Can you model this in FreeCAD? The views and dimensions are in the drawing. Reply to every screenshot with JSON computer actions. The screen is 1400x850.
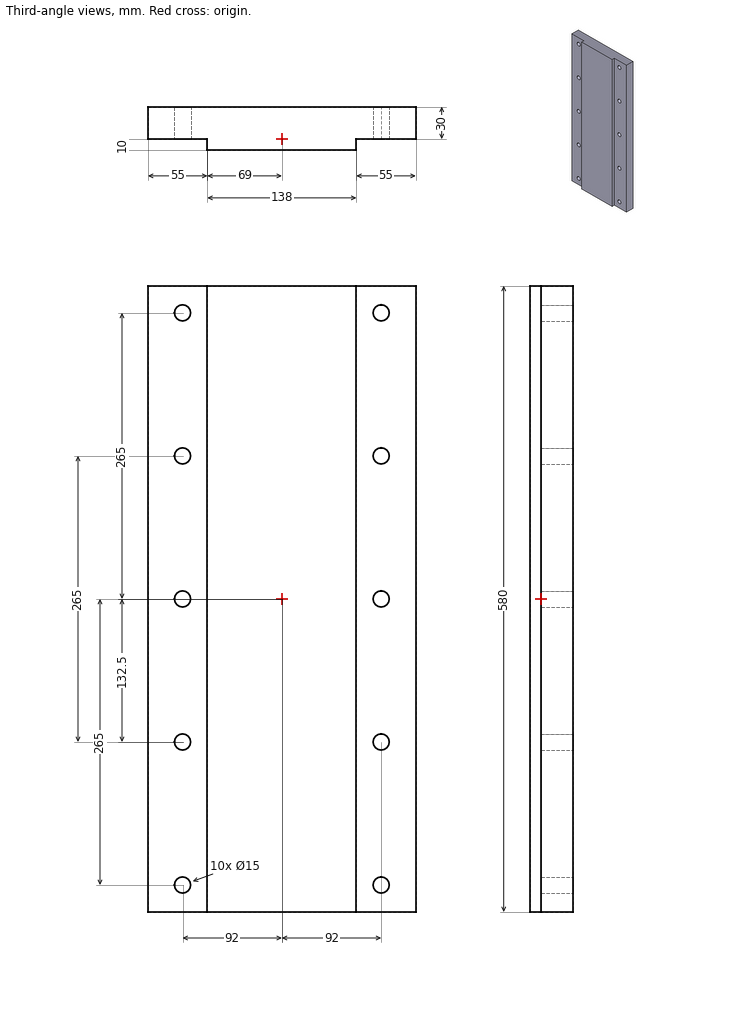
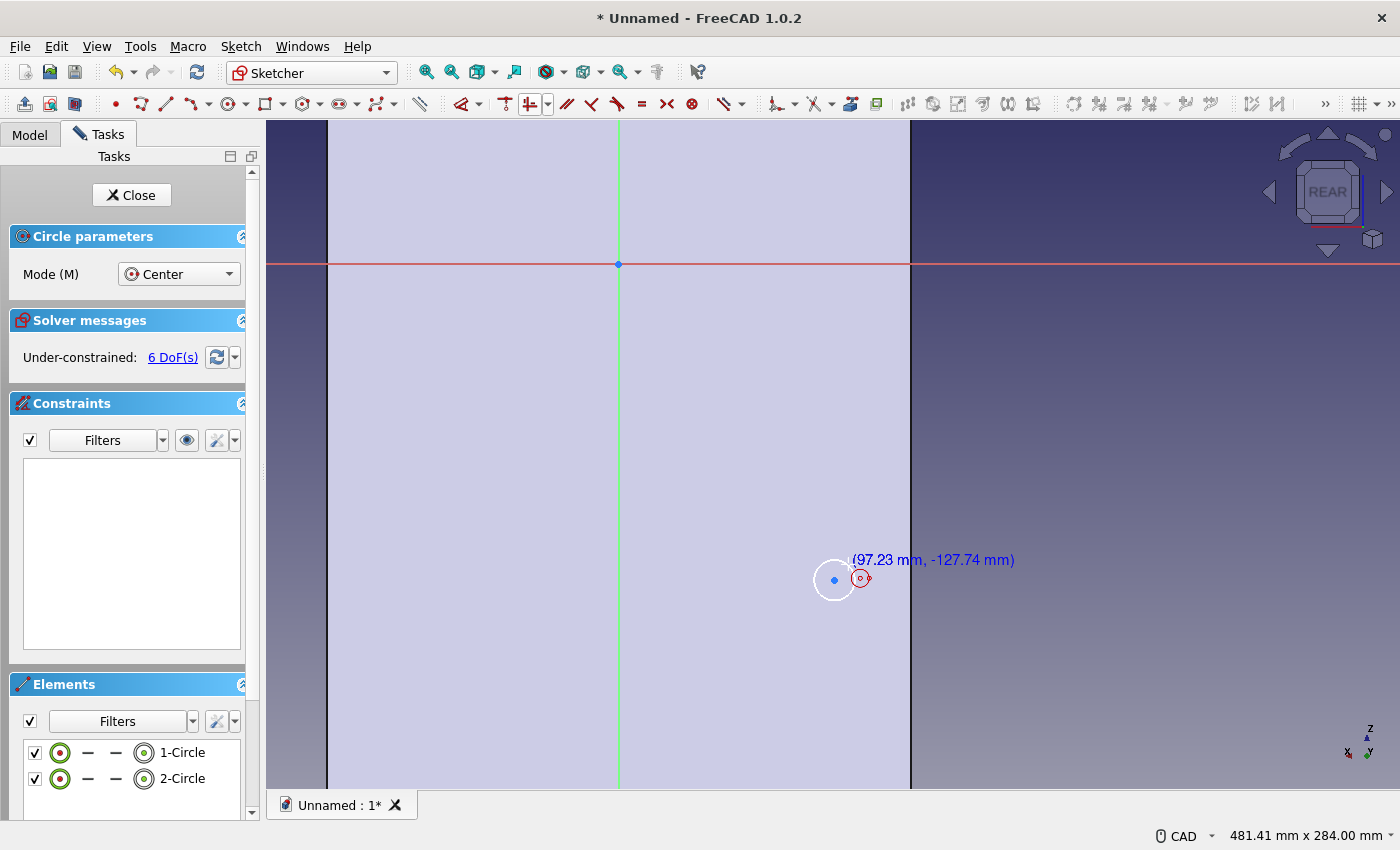
{"action": "scroll", "coordinate": [836, 264], "scroll_direction": "up", "scroll_amount": 2}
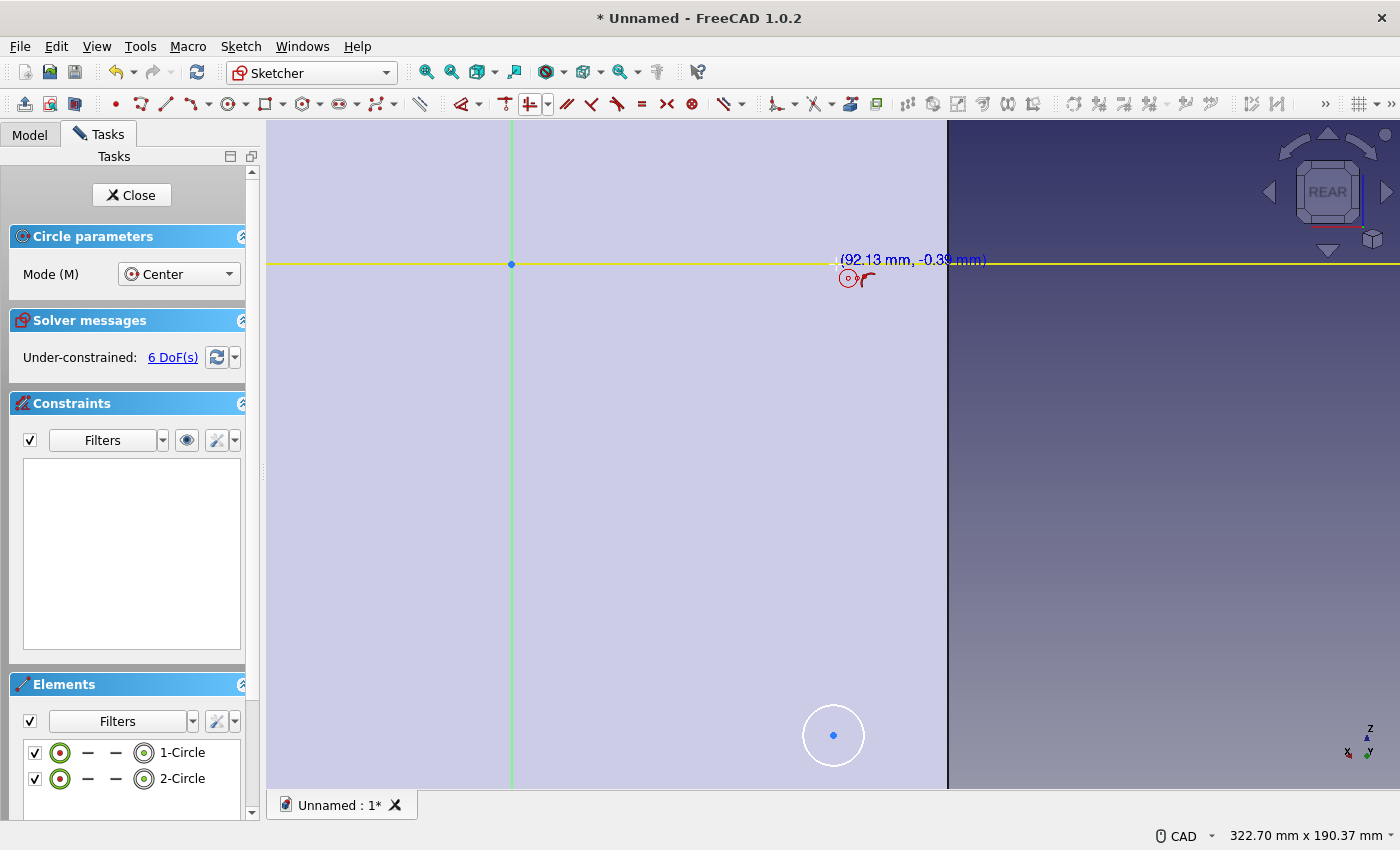
{"action": "scroll", "coordinate": [847, 517], "scroll_direction": "down", "scroll_amount": 7}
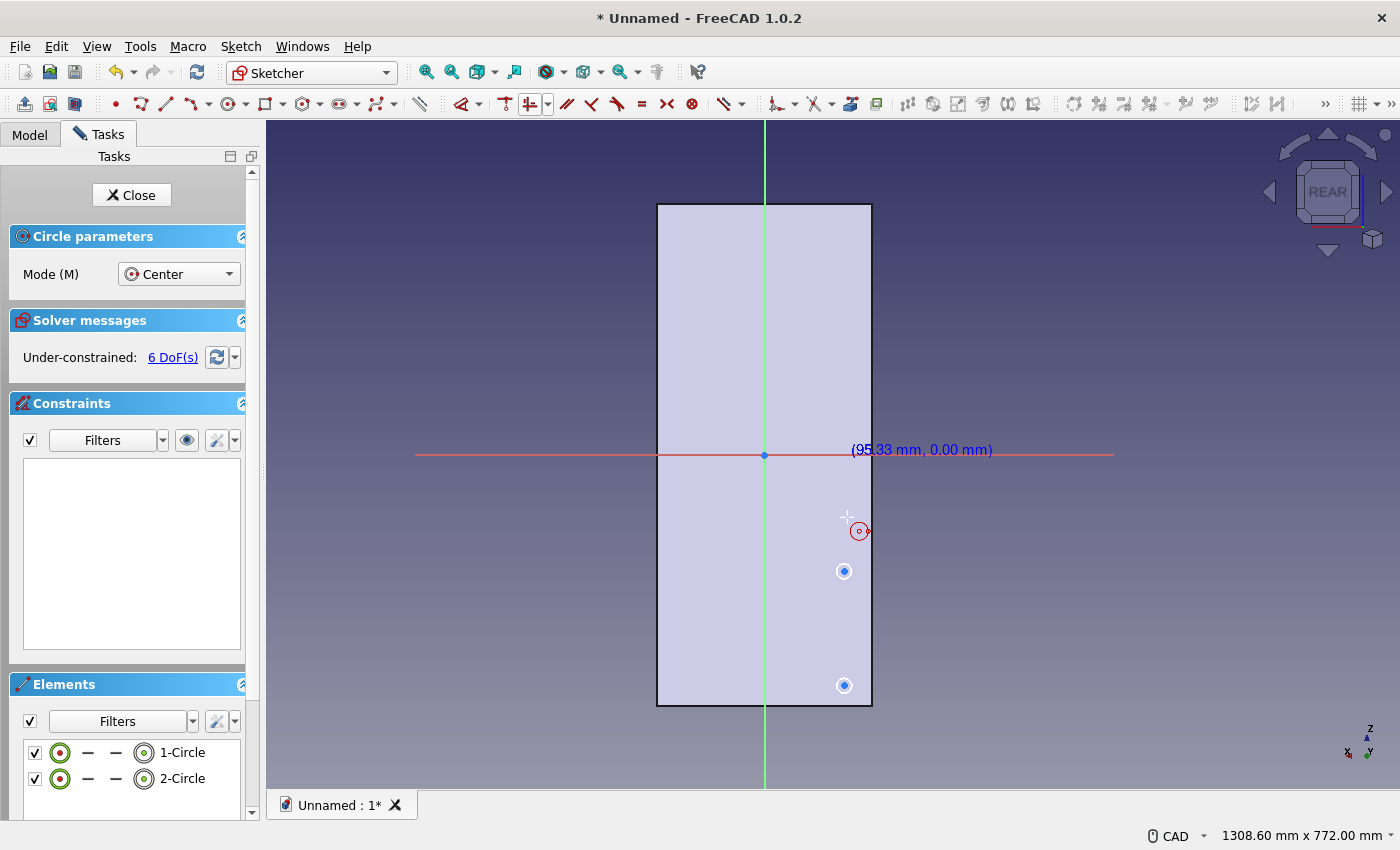
{"action": "left_click", "coordinate": [844, 455]}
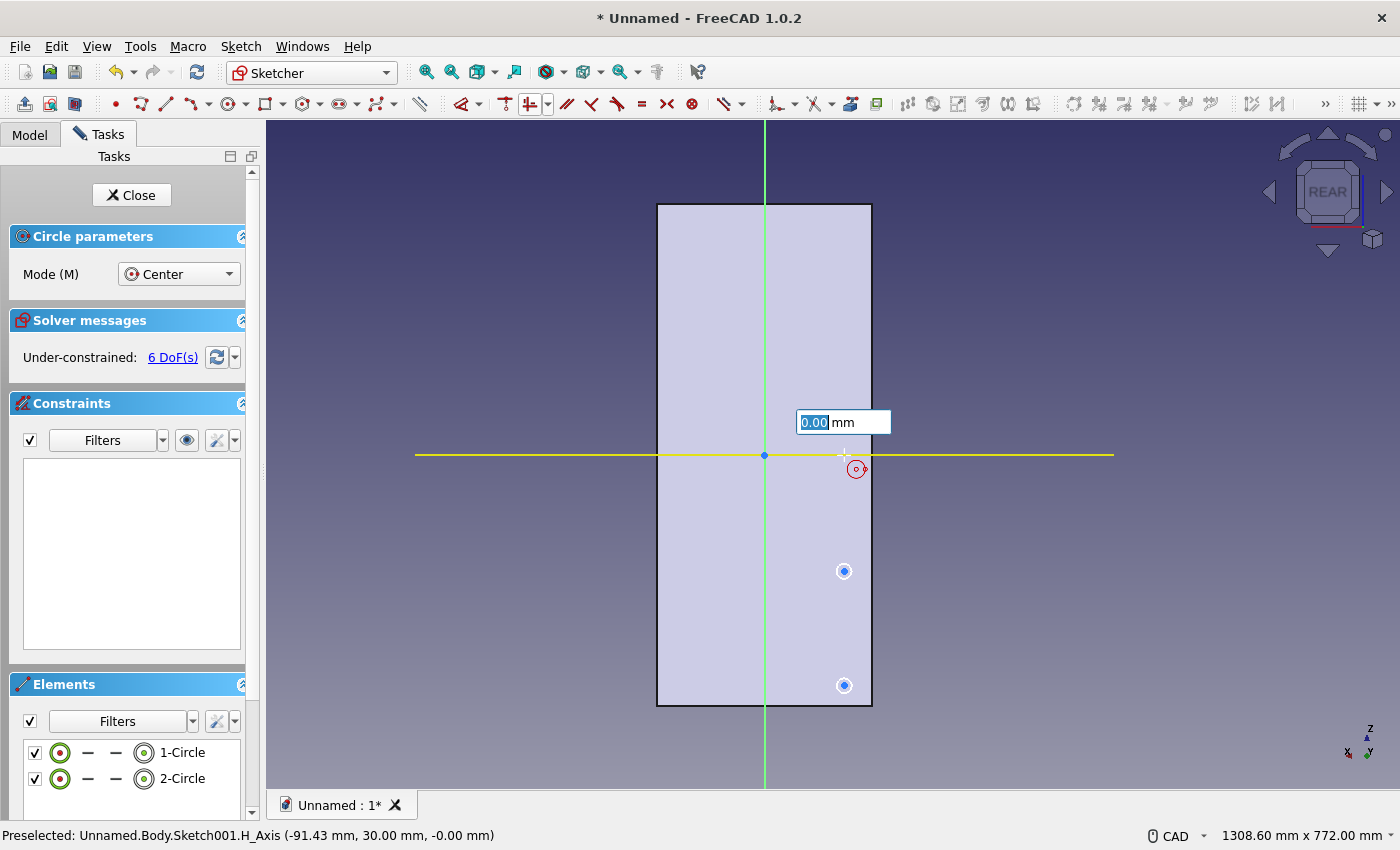
{"action": "scroll", "coordinate": [842, 461], "scroll_direction": "up", "scroll_amount": 5}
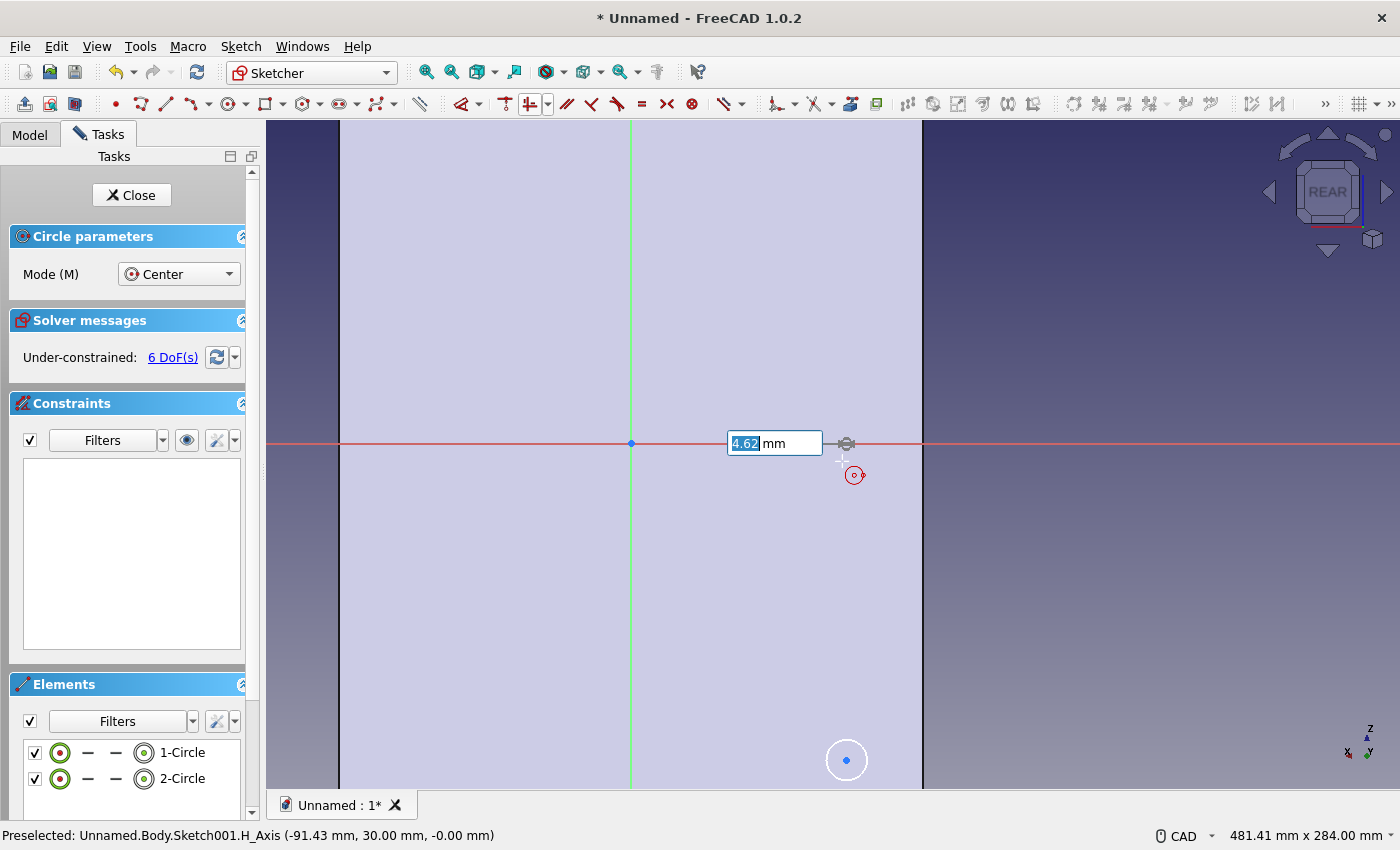
{"action": "left_click", "coordinate": [842, 461]}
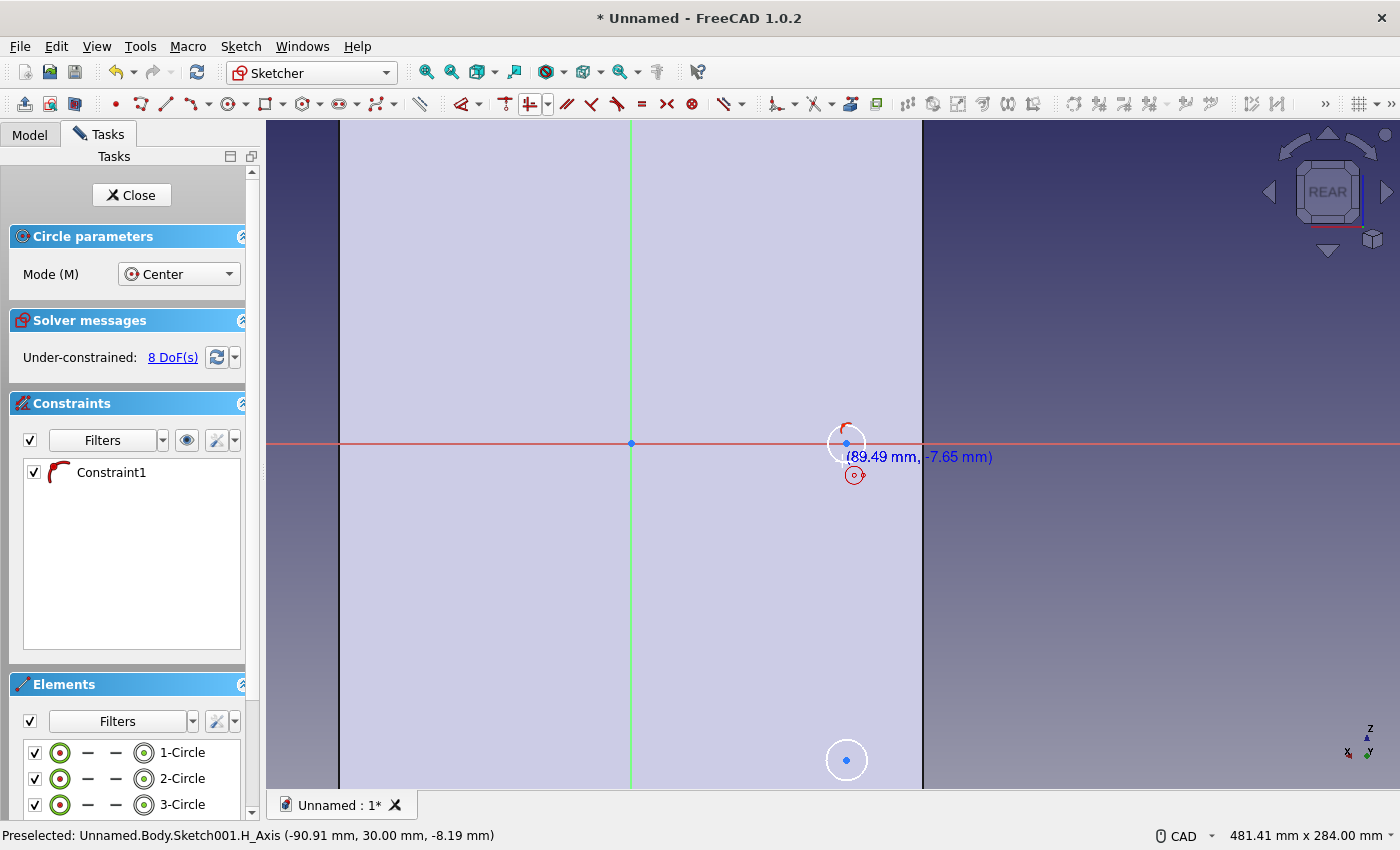
{"action": "scroll", "coordinate": [842, 461], "scroll_direction": "down", "scroll_amount": 5}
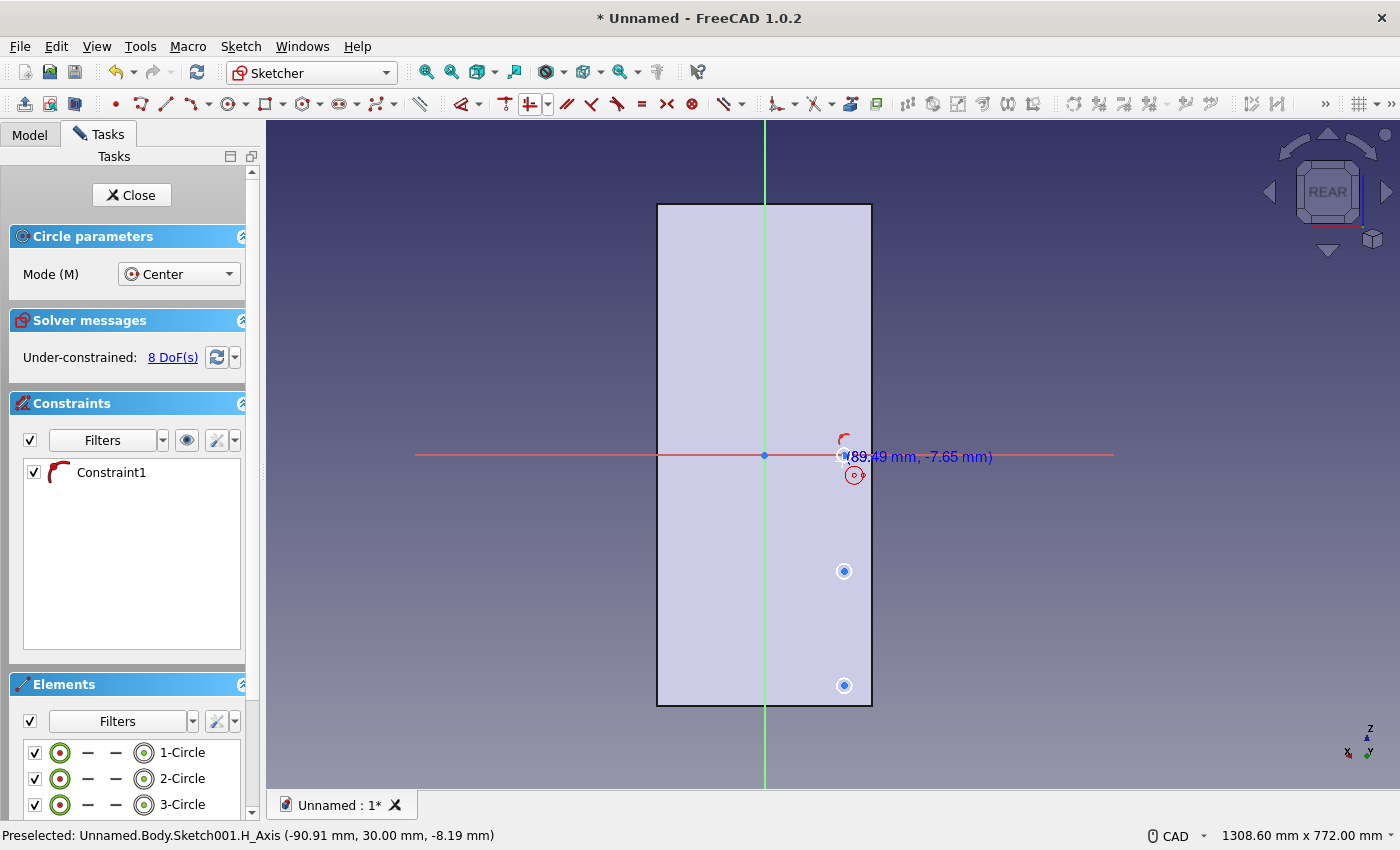
{"action": "scroll", "coordinate": [844, 340], "scroll_direction": "up", "scroll_amount": 7}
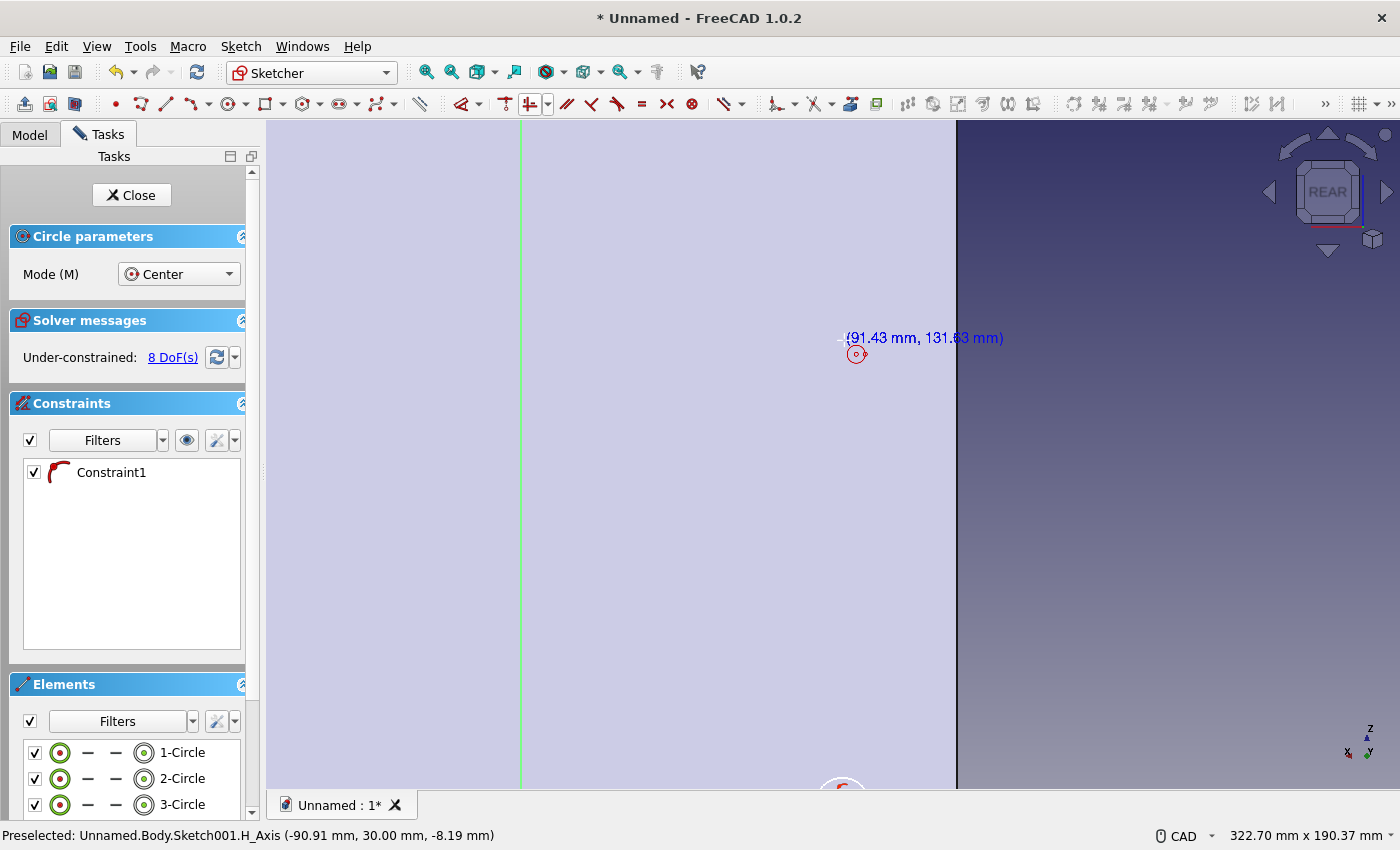
{"action": "scroll", "coordinate": [844, 340], "scroll_direction": "down", "scroll_amount": 7}